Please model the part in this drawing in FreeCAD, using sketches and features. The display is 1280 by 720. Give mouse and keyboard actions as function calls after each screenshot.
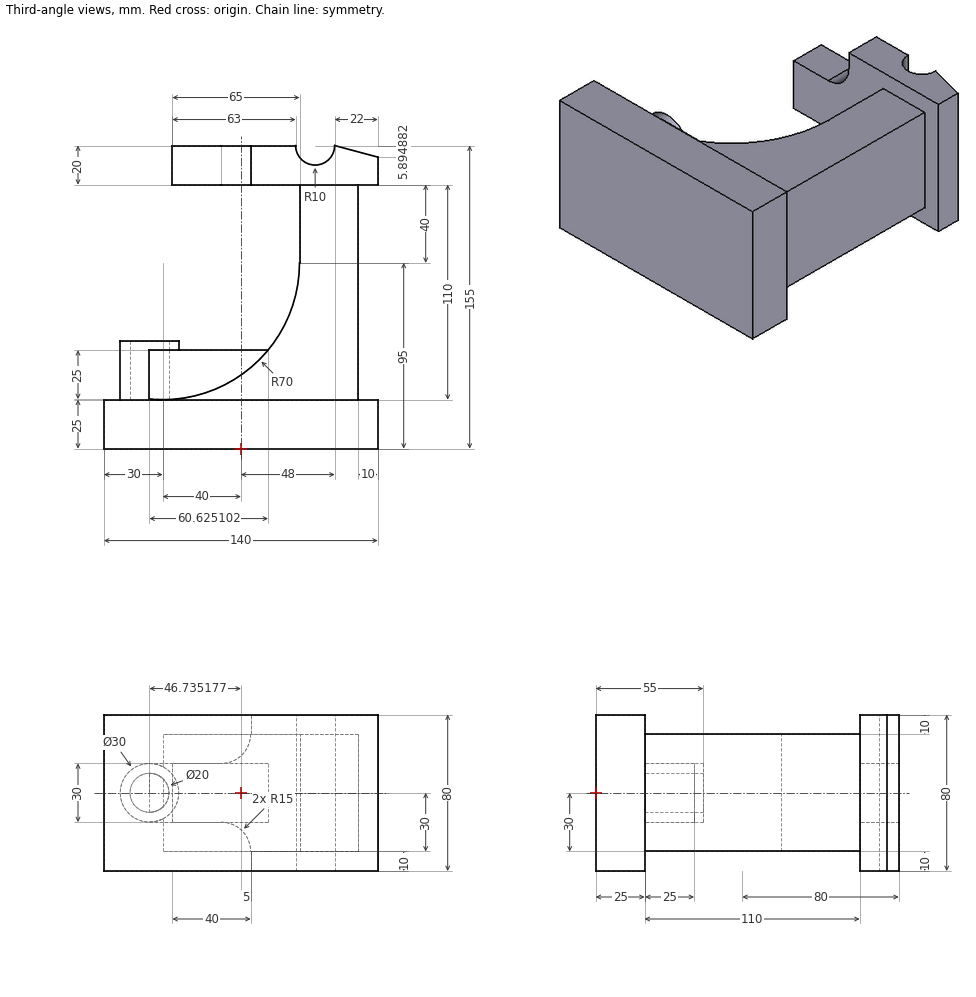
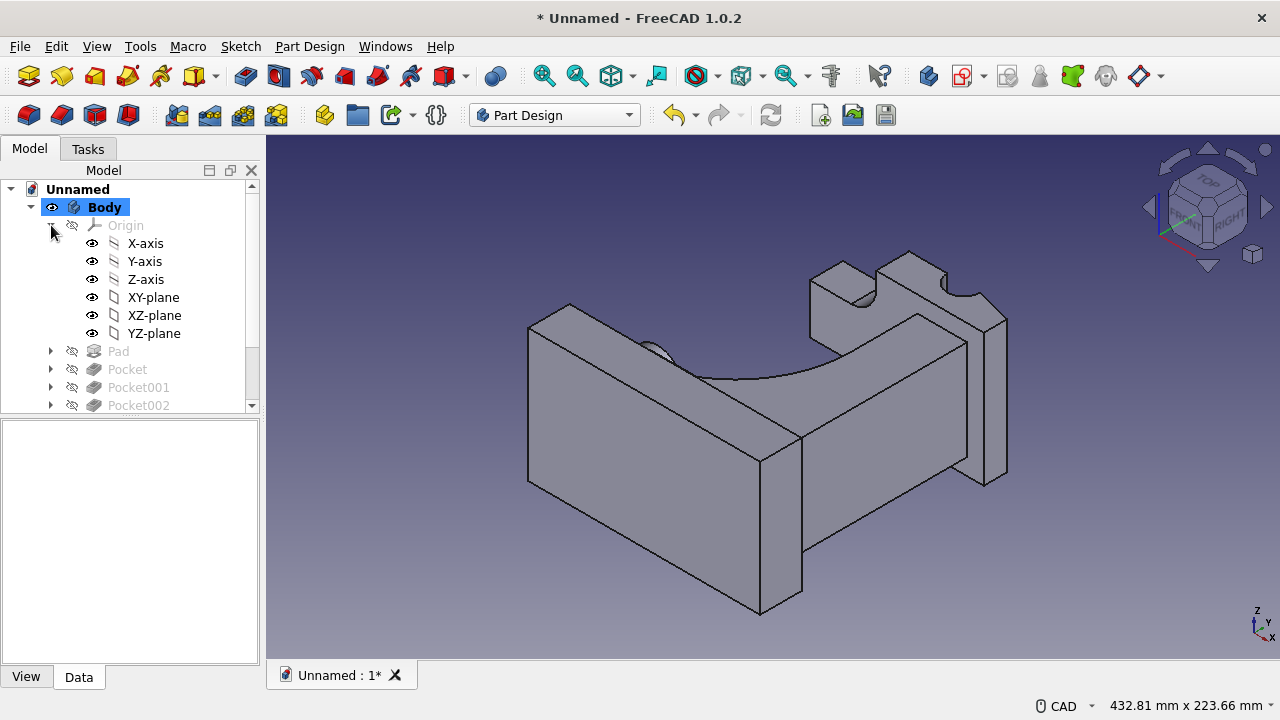
click(137, 315)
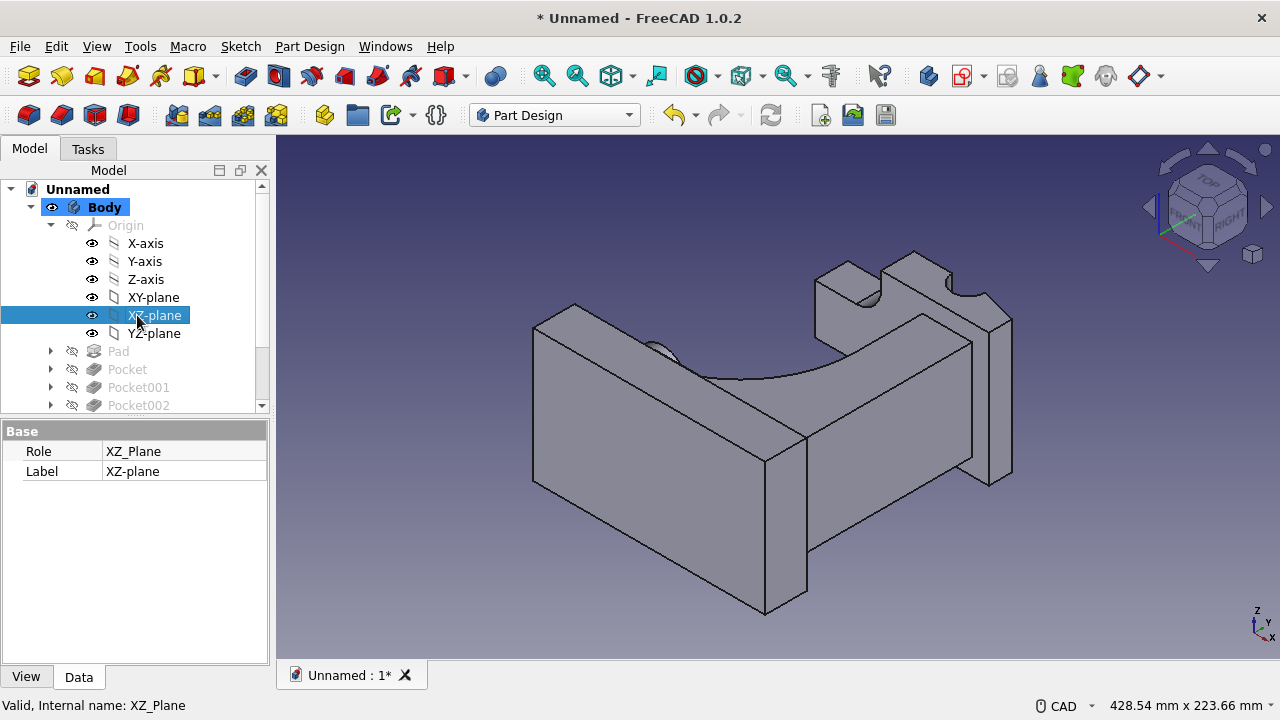
click(1138, 76)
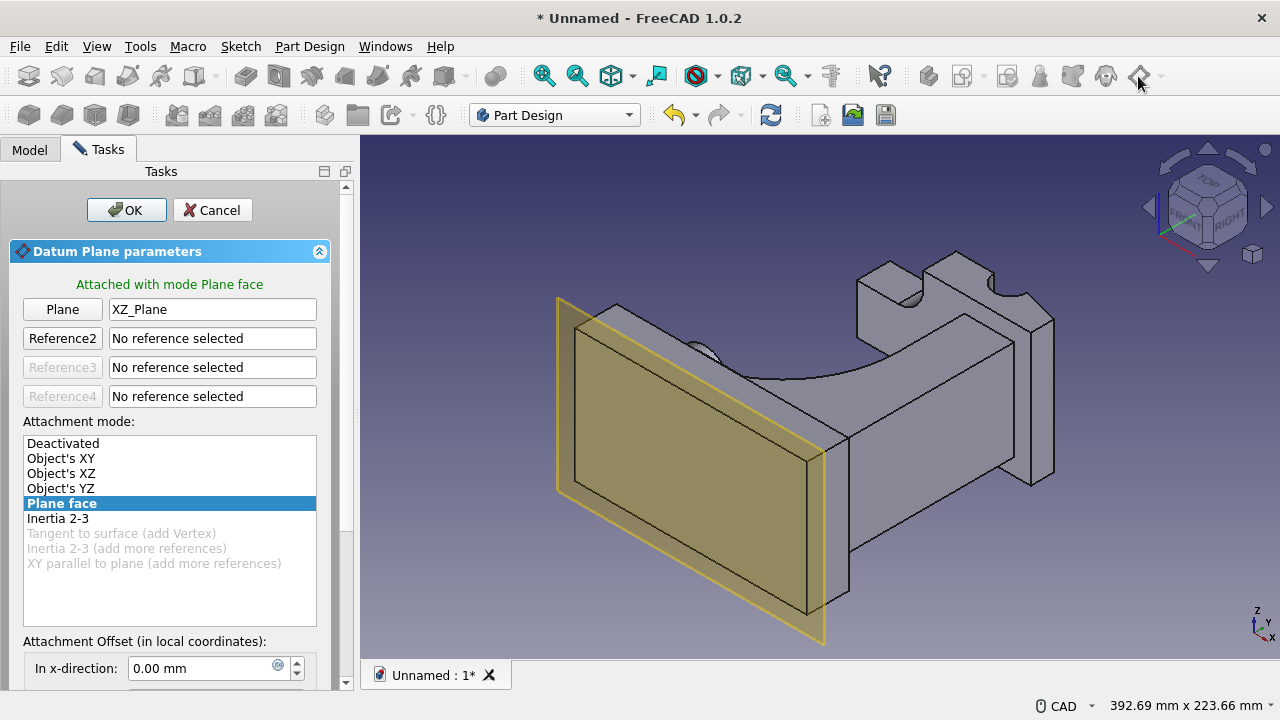
scroll(346, 436, down, 2)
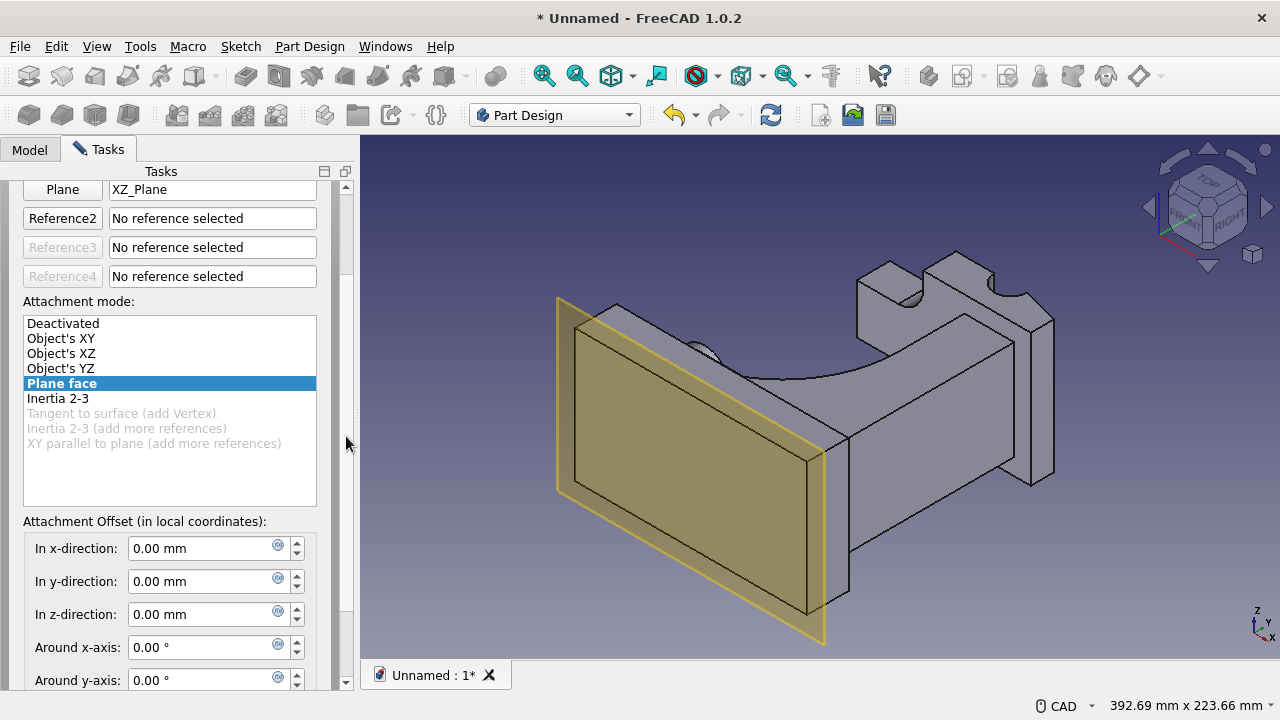
triple_click(210, 614)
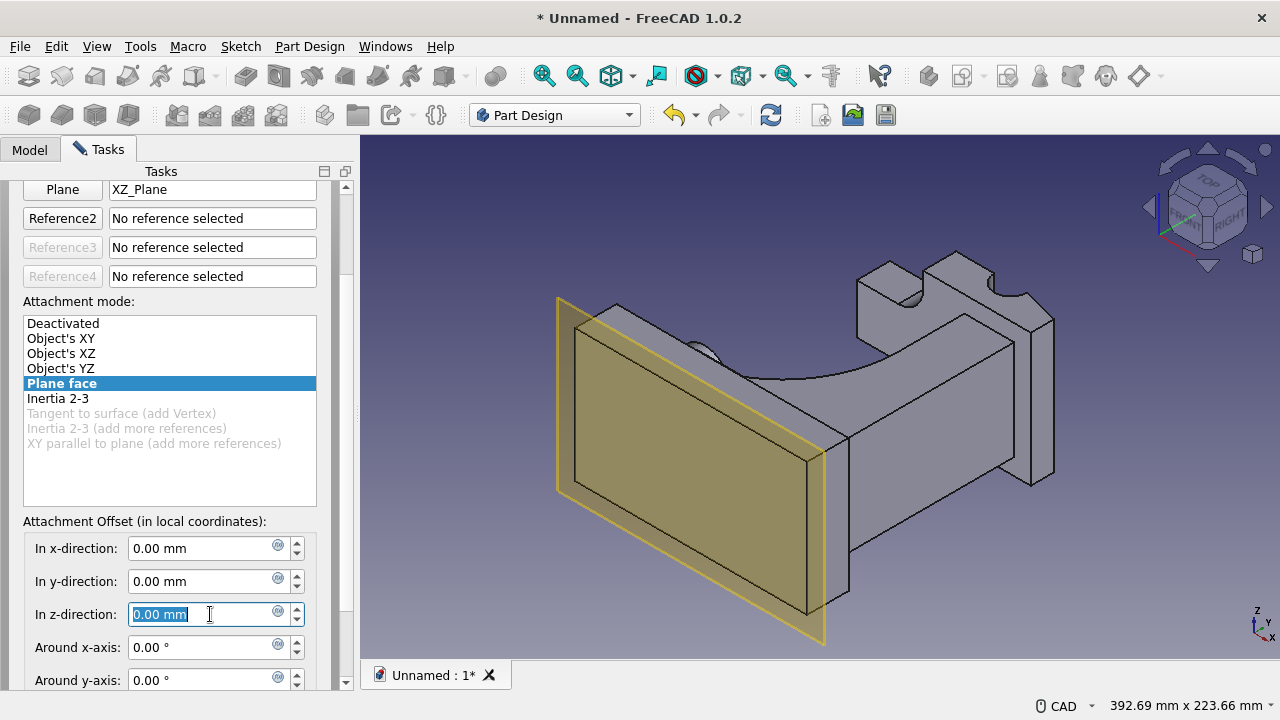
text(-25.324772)
key(Tab)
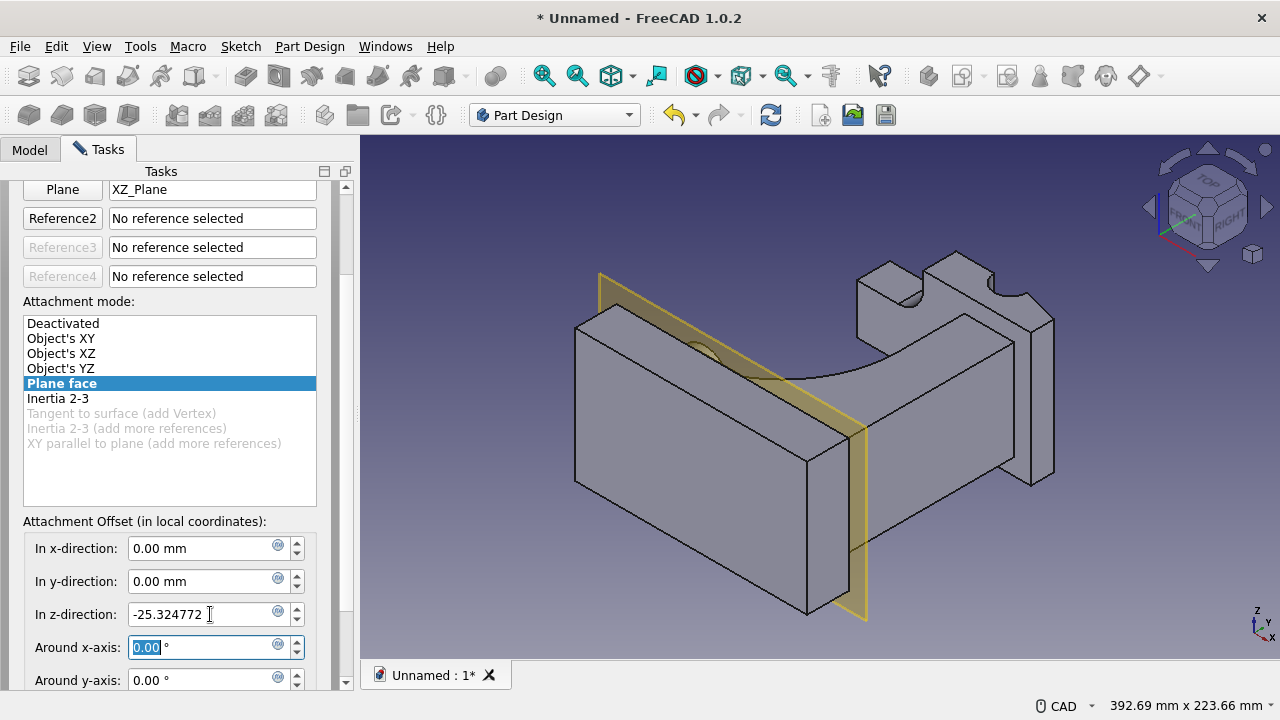
scroll(346, 436, up, 3)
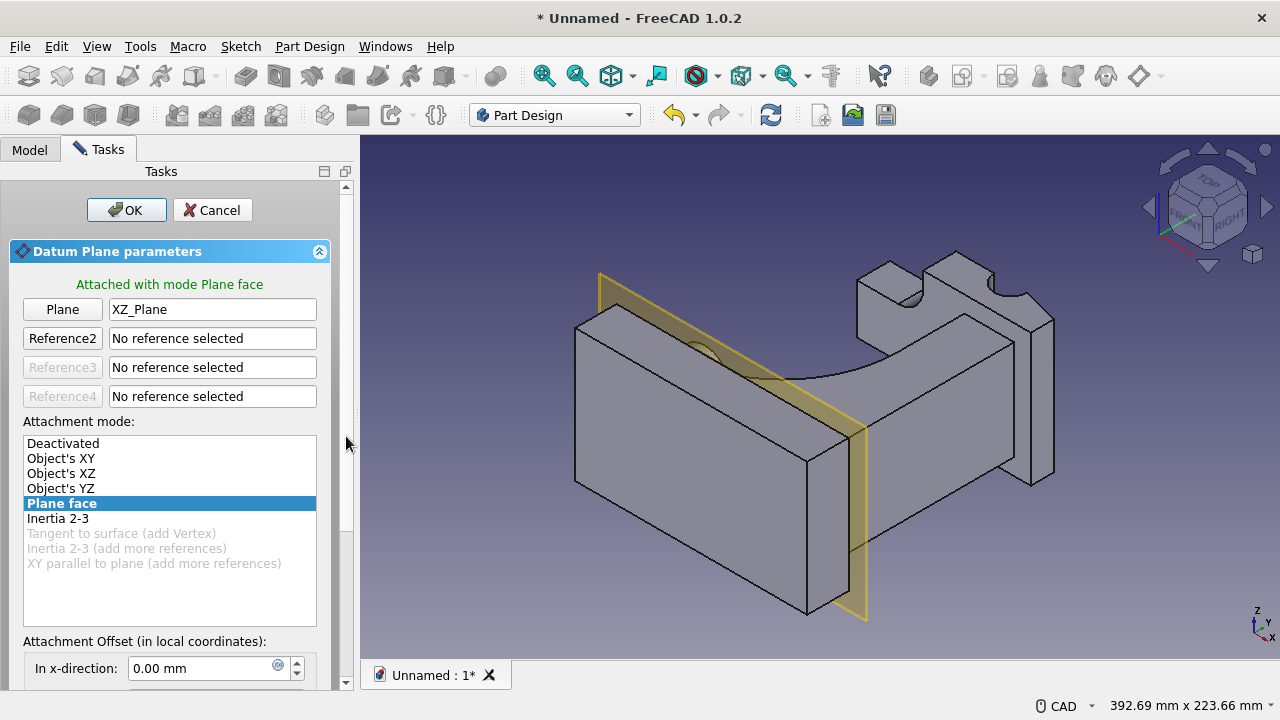
click(127, 210)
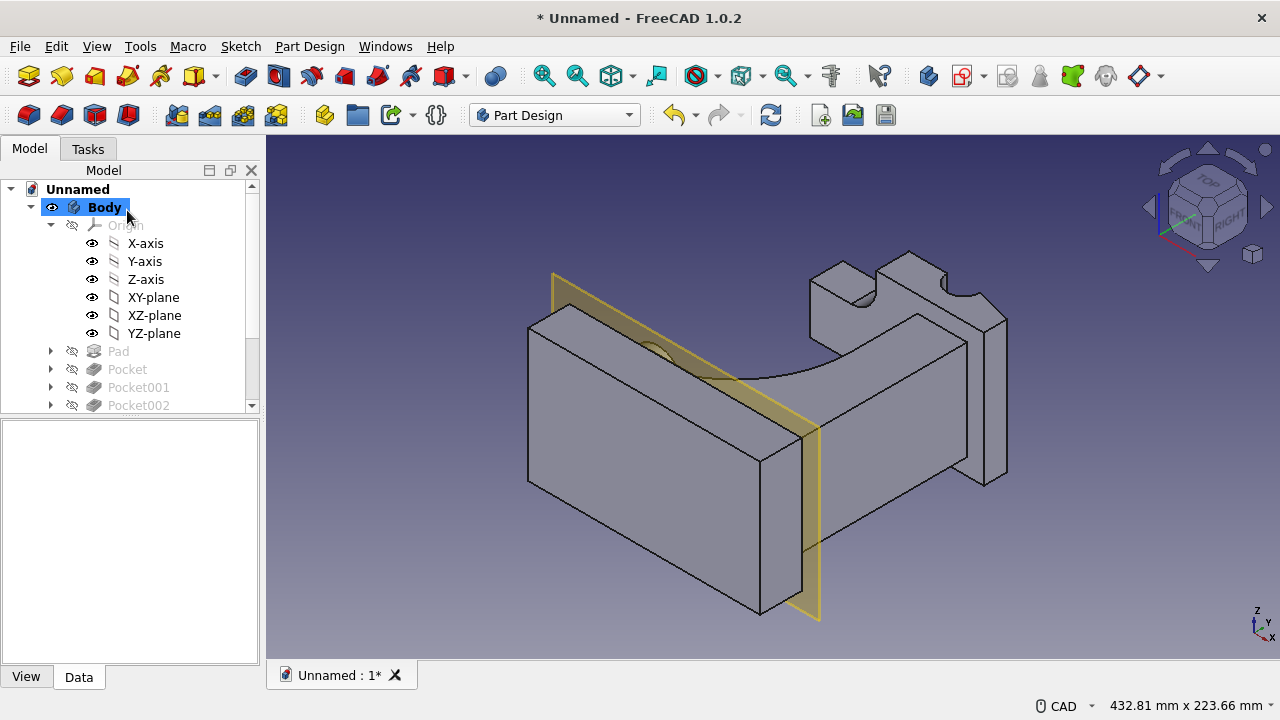
scroll(101, 293, down, 3)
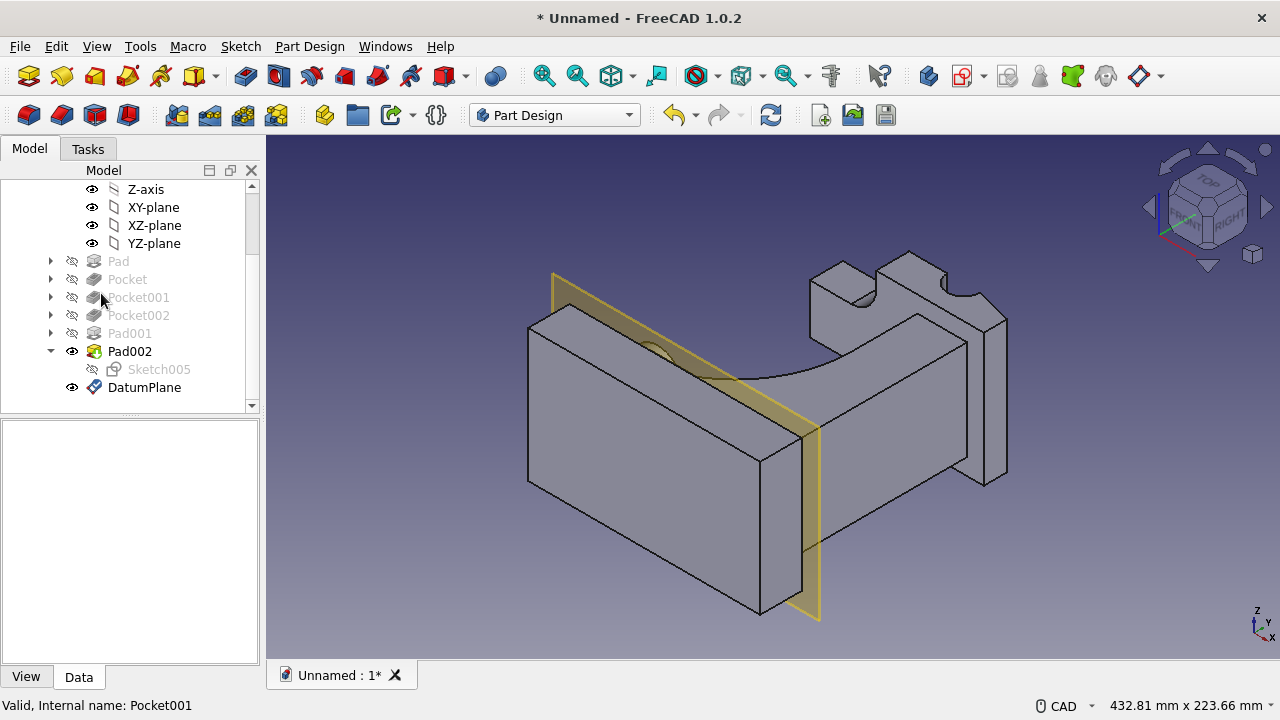
click(117, 387)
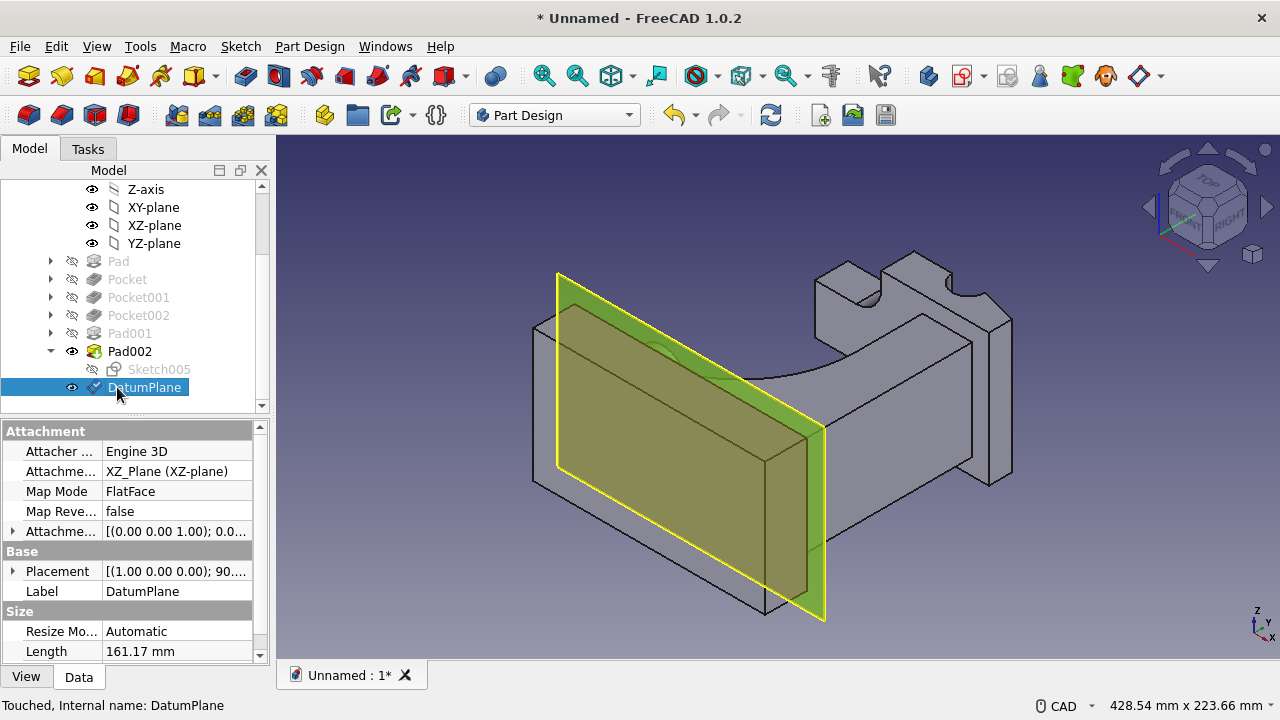
click(962, 76)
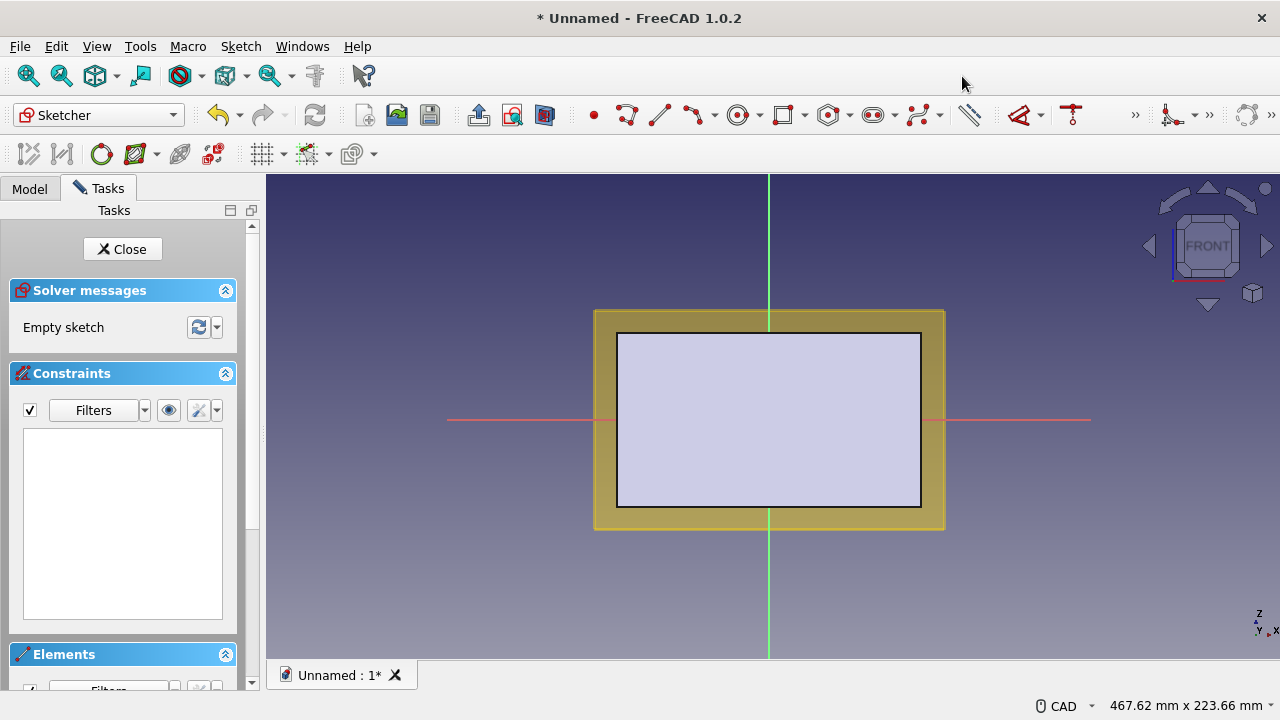
click(545, 116)